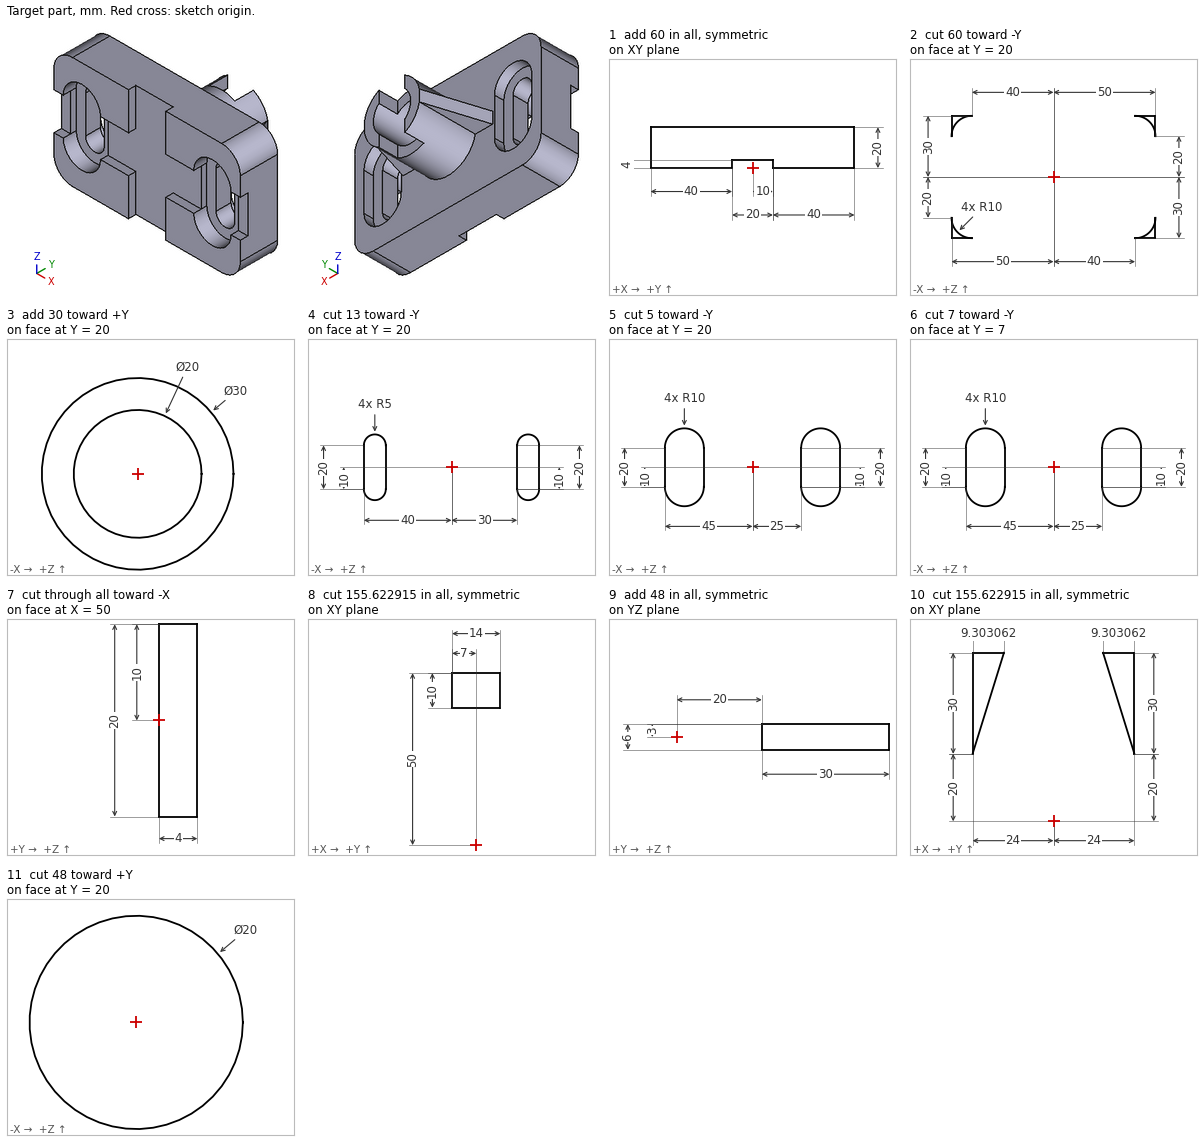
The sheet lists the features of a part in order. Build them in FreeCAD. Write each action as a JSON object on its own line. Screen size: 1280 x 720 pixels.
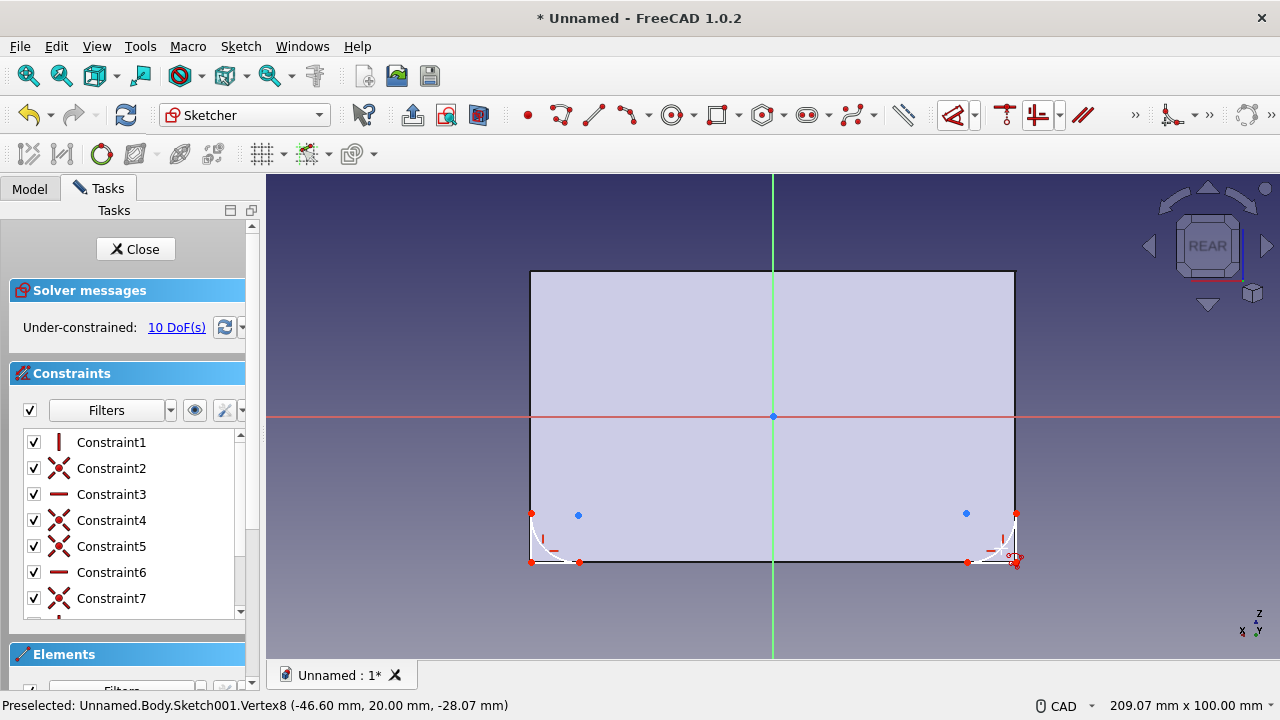
{"action": "left_click", "coordinate": [1016, 319]}
{"action": "left_click", "coordinate": [1016, 271]}
{"action": "left_click", "coordinate": [967, 271]}
{"action": "right_click", "coordinate": [967, 271]}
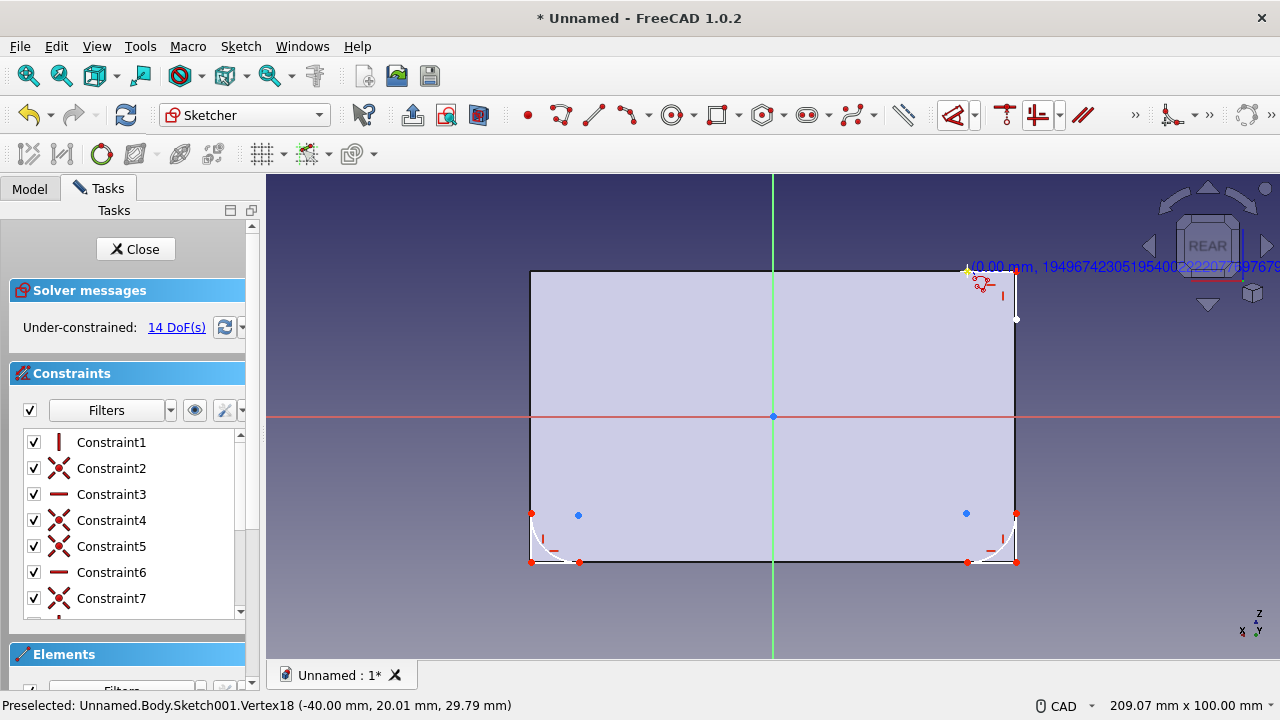
{"action": "left_click", "coordinate": [626, 116]}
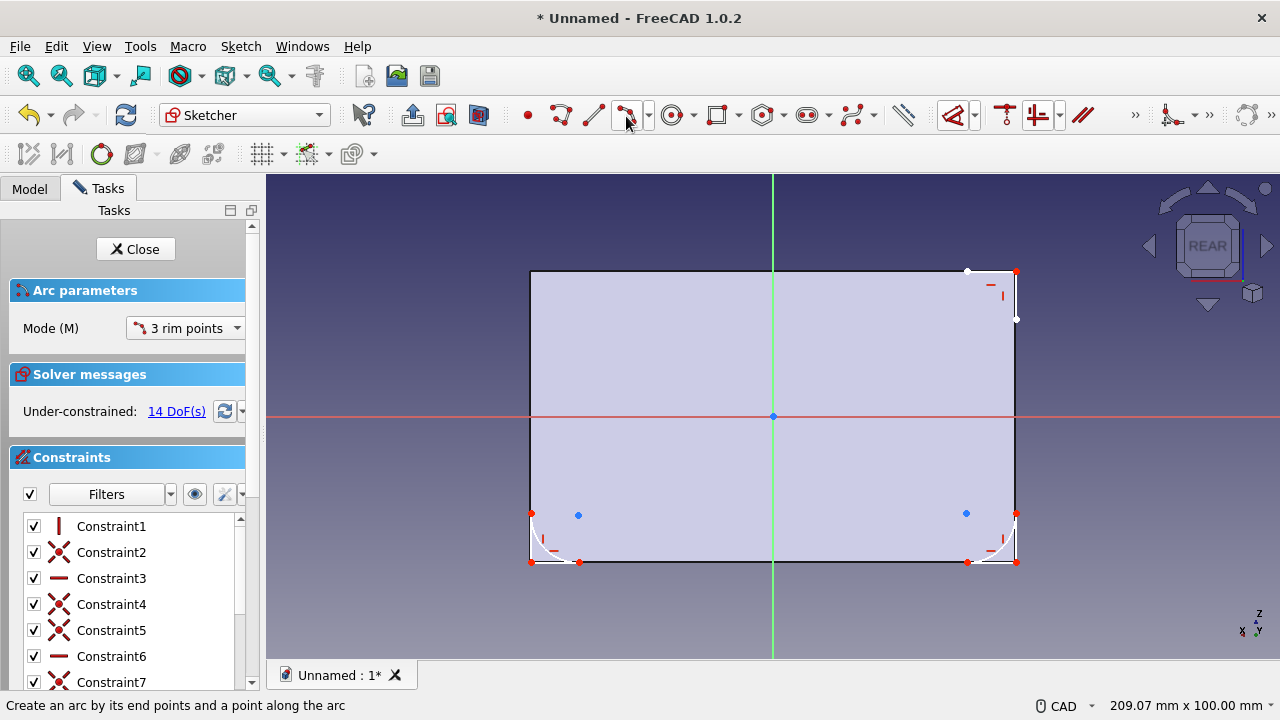
{"action": "left_click", "coordinate": [967, 272]}
{"action": "left_click", "coordinate": [1016, 320]}
{"action": "left_click", "coordinate": [1001, 285]}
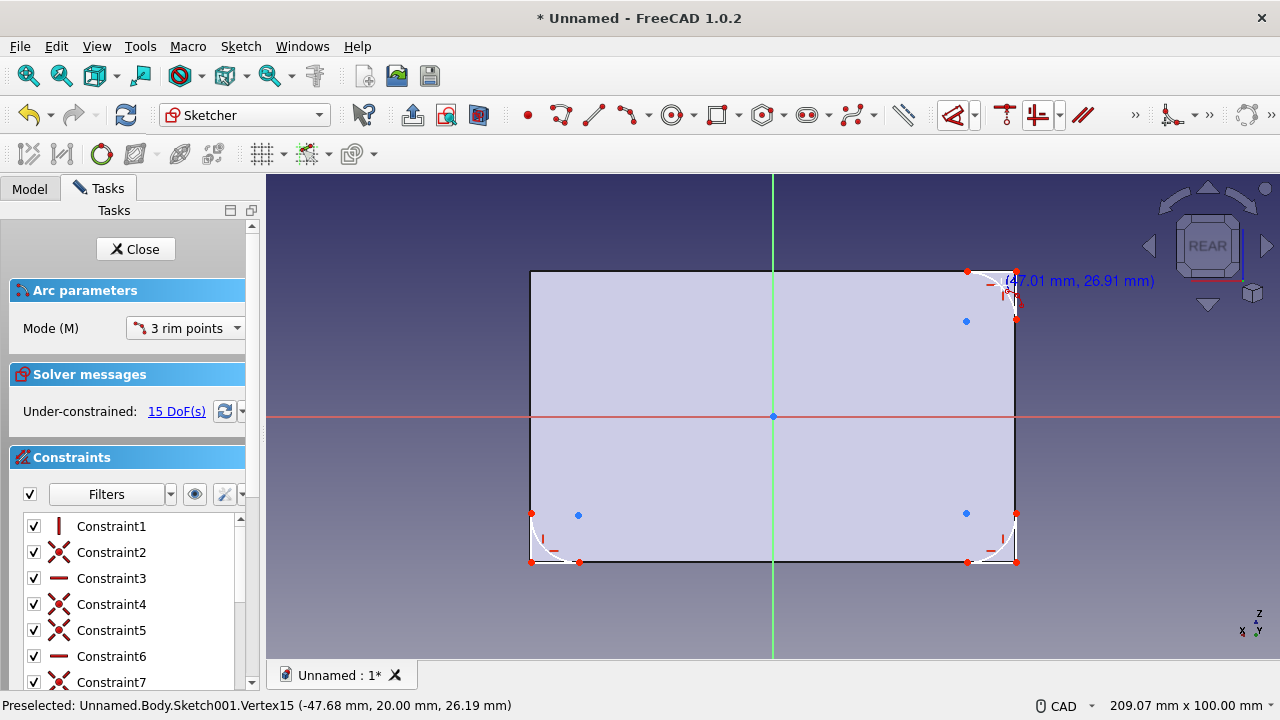
{"action": "left_click", "coordinate": [561, 116]}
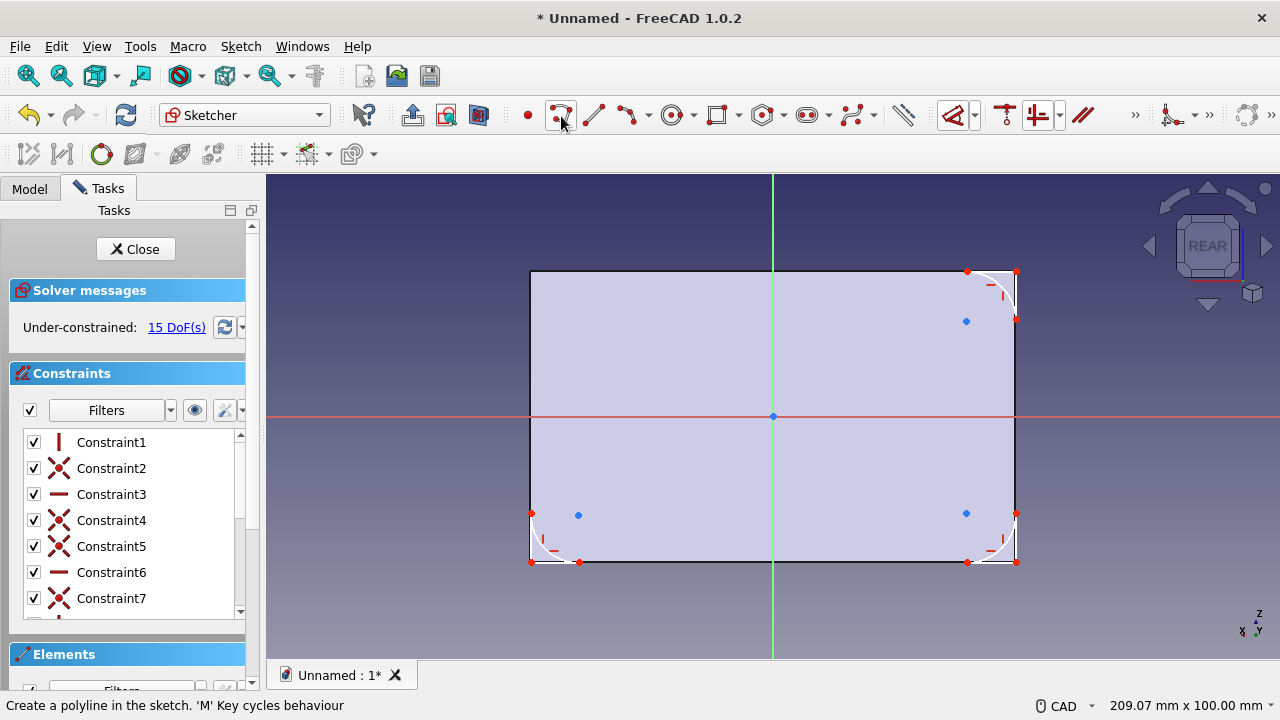
{"action": "left_click", "coordinate": [579, 271]}
{"action": "left_click", "coordinate": [531, 271]}
{"action": "left_click", "coordinate": [531, 319]}
{"action": "right_click", "coordinate": [531, 319]}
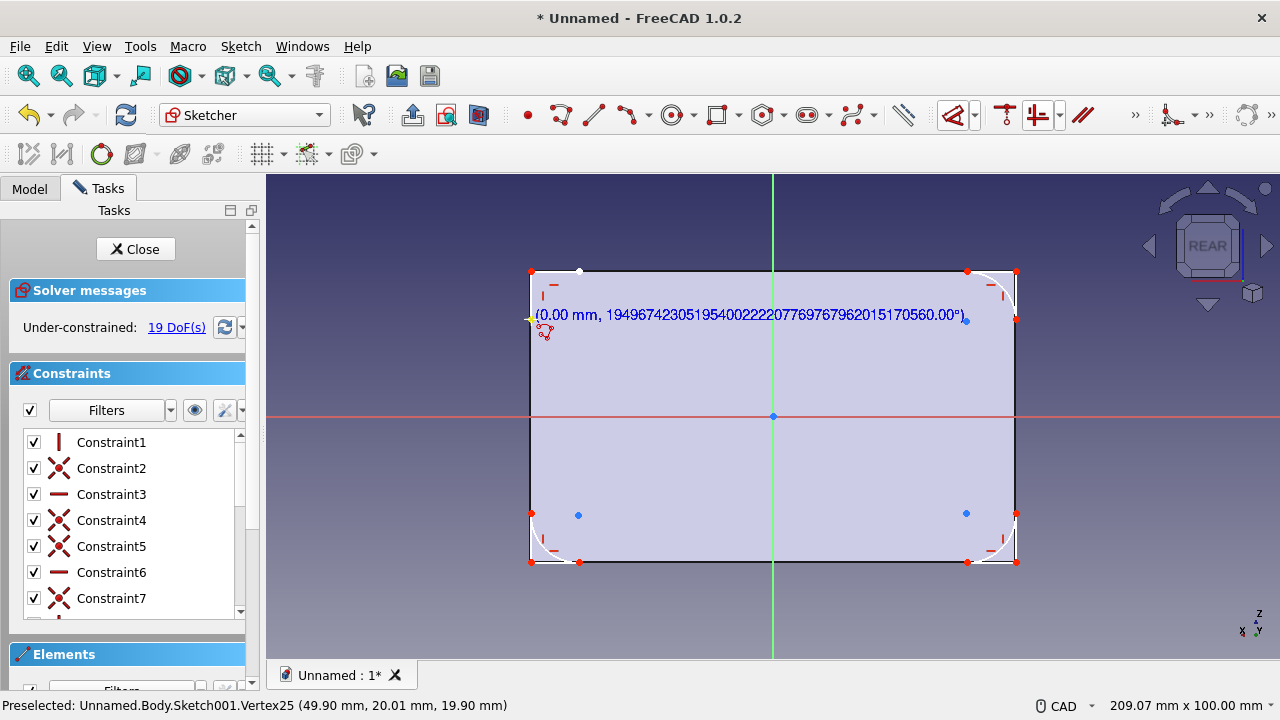
{"action": "left_click", "coordinate": [626, 116]}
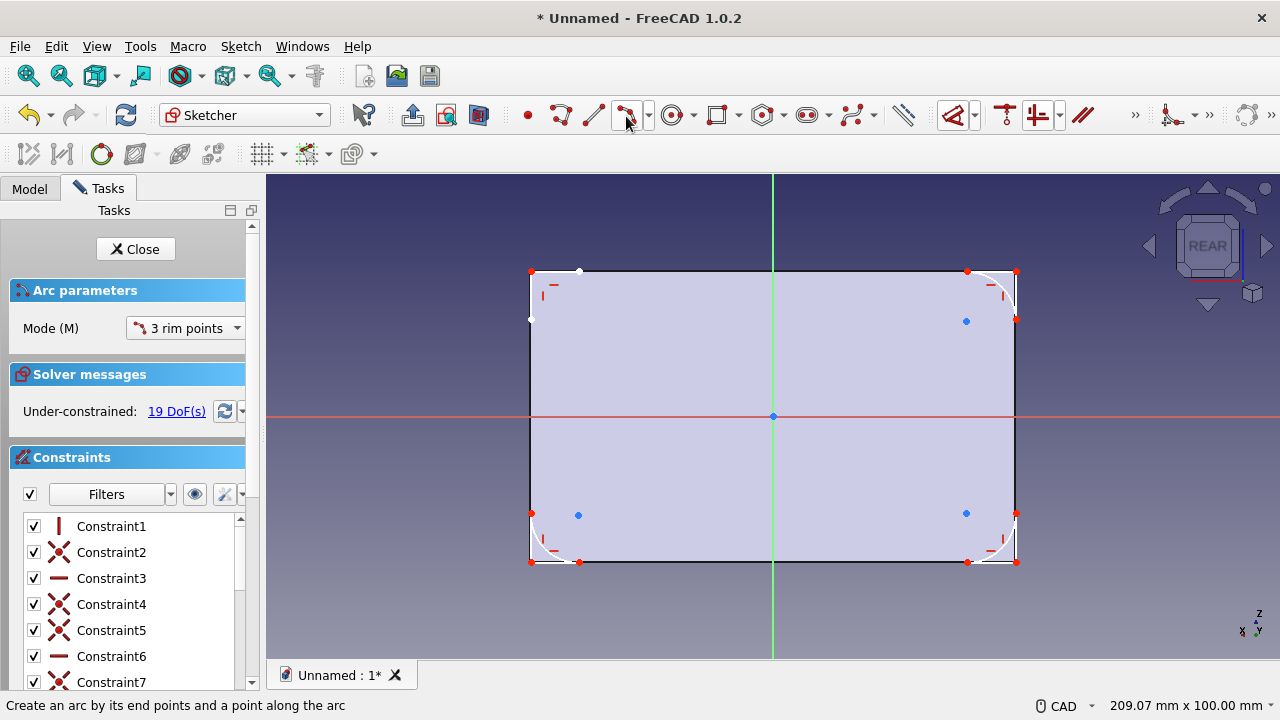
{"action": "left_click", "coordinate": [531, 320]}
{"action": "left_click", "coordinate": [579, 272]}
{"action": "left_click", "coordinate": [545, 285]}
{"action": "key", "text": "Escape"}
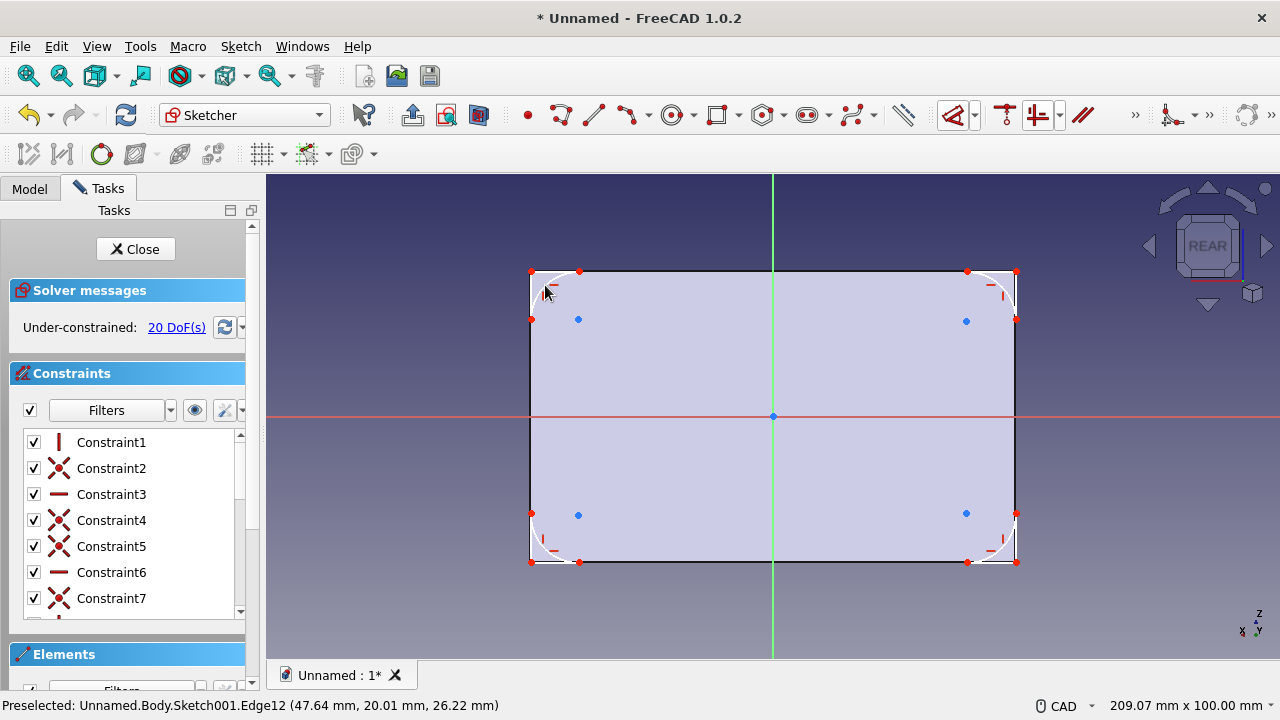
{"action": "scroll", "coordinate": [531, 548], "scroll_direction": "up", "scroll_amount": 2}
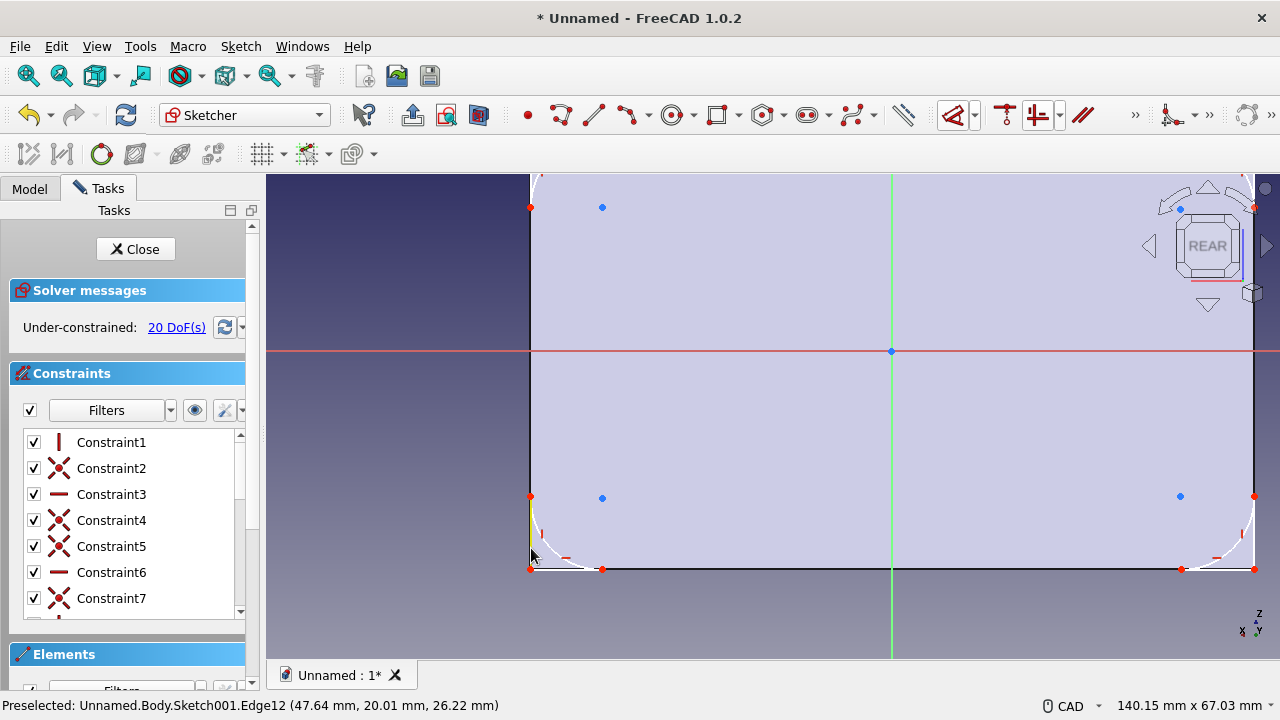
{"action": "left_click", "coordinate": [531, 548]}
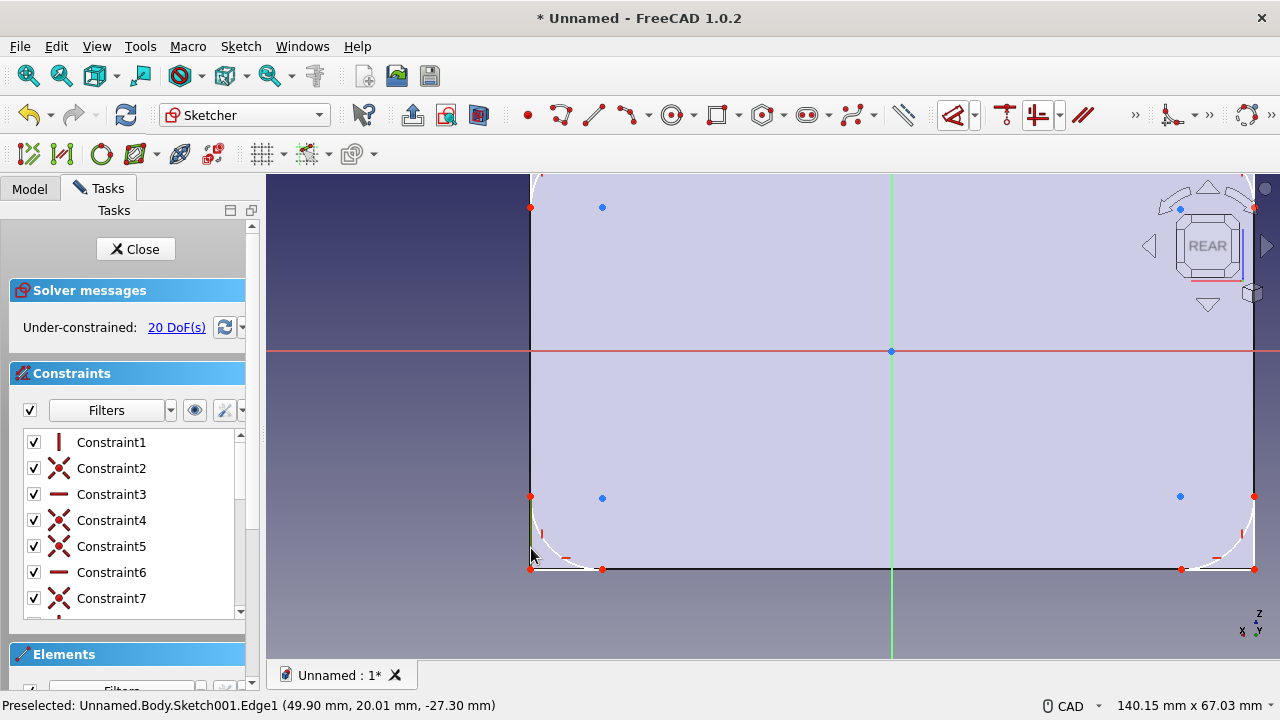
{"action": "left_click", "coordinate": [551, 549]}